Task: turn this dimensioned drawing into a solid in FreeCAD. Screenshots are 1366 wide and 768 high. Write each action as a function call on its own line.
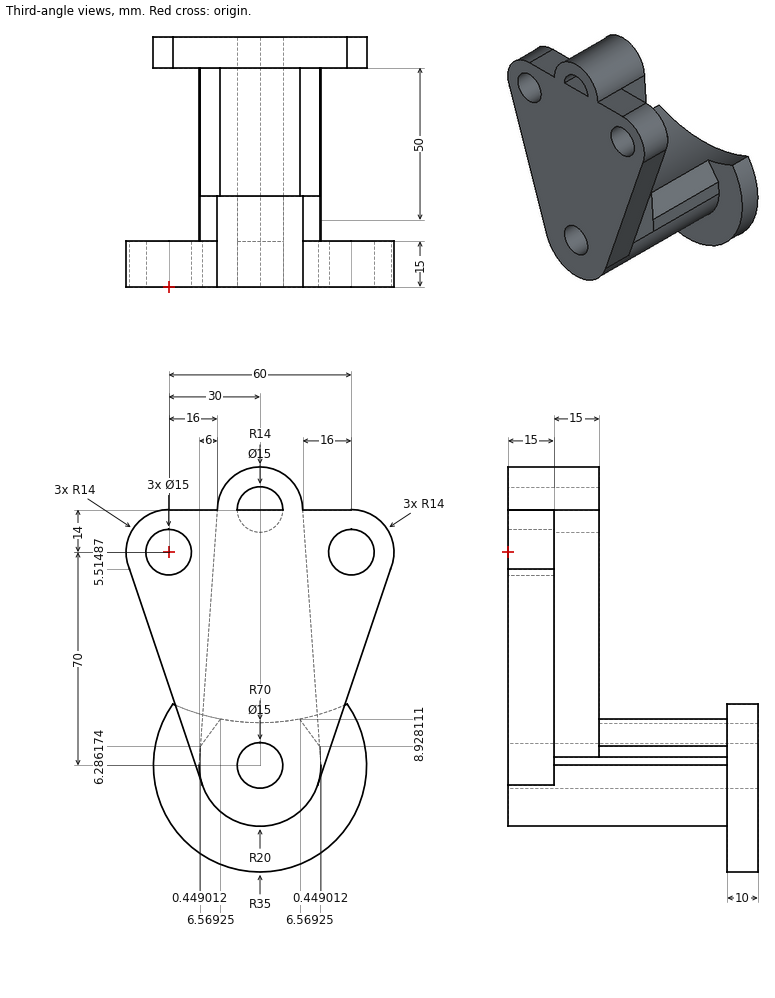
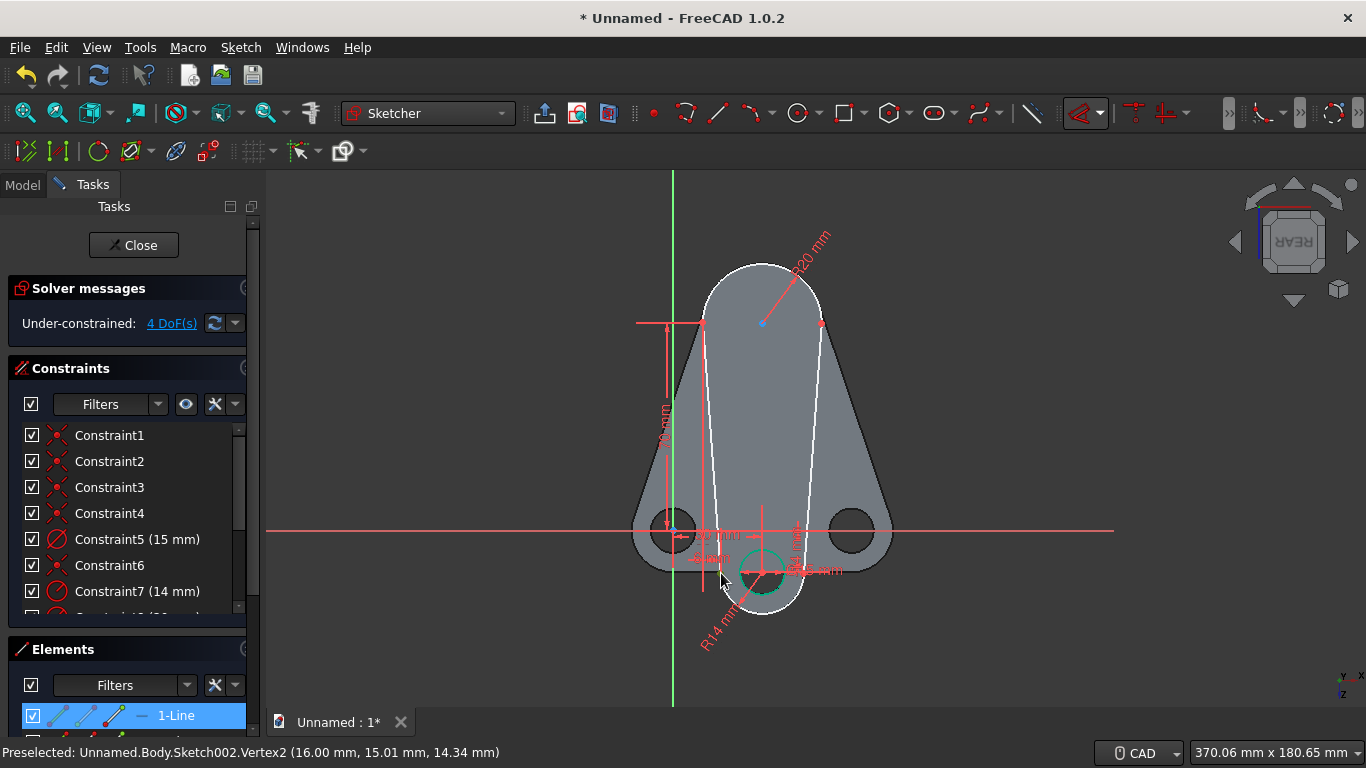
key(i)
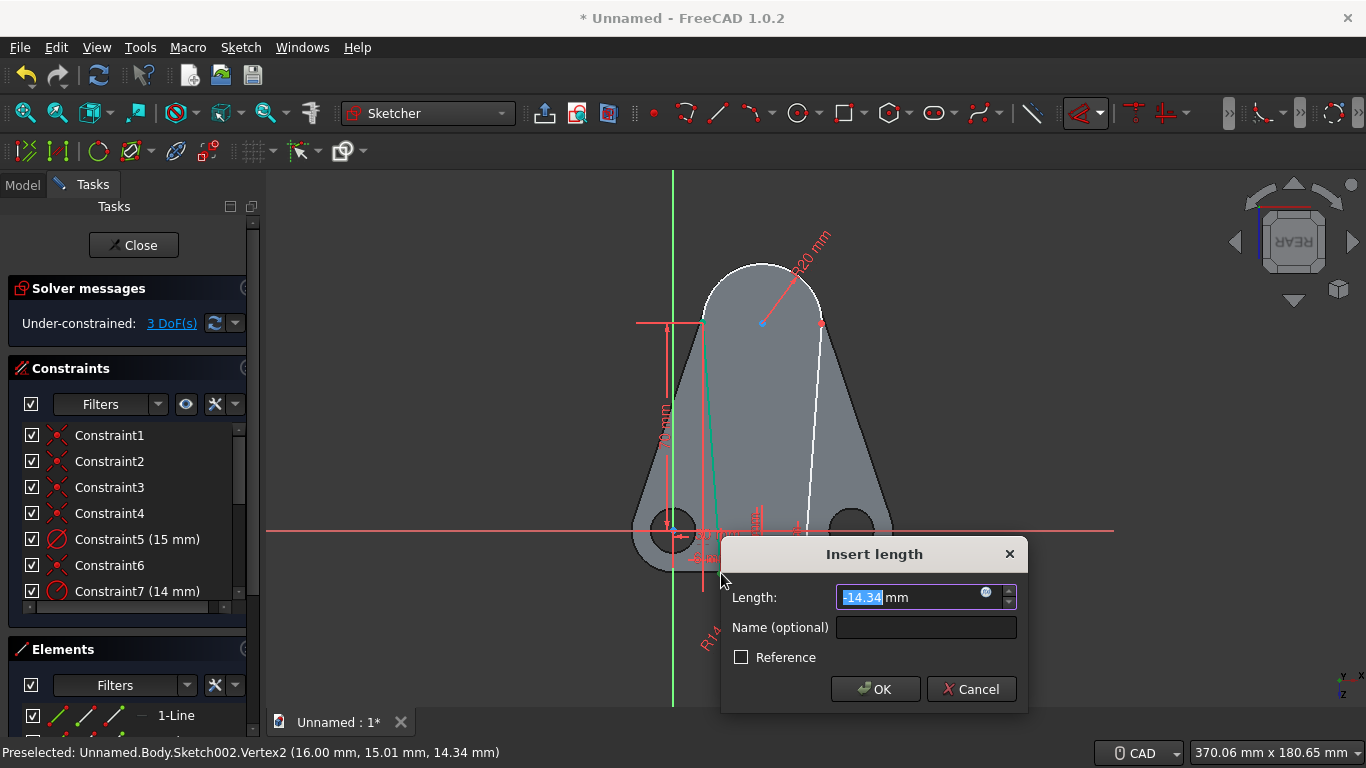
text(-14)
key(Return)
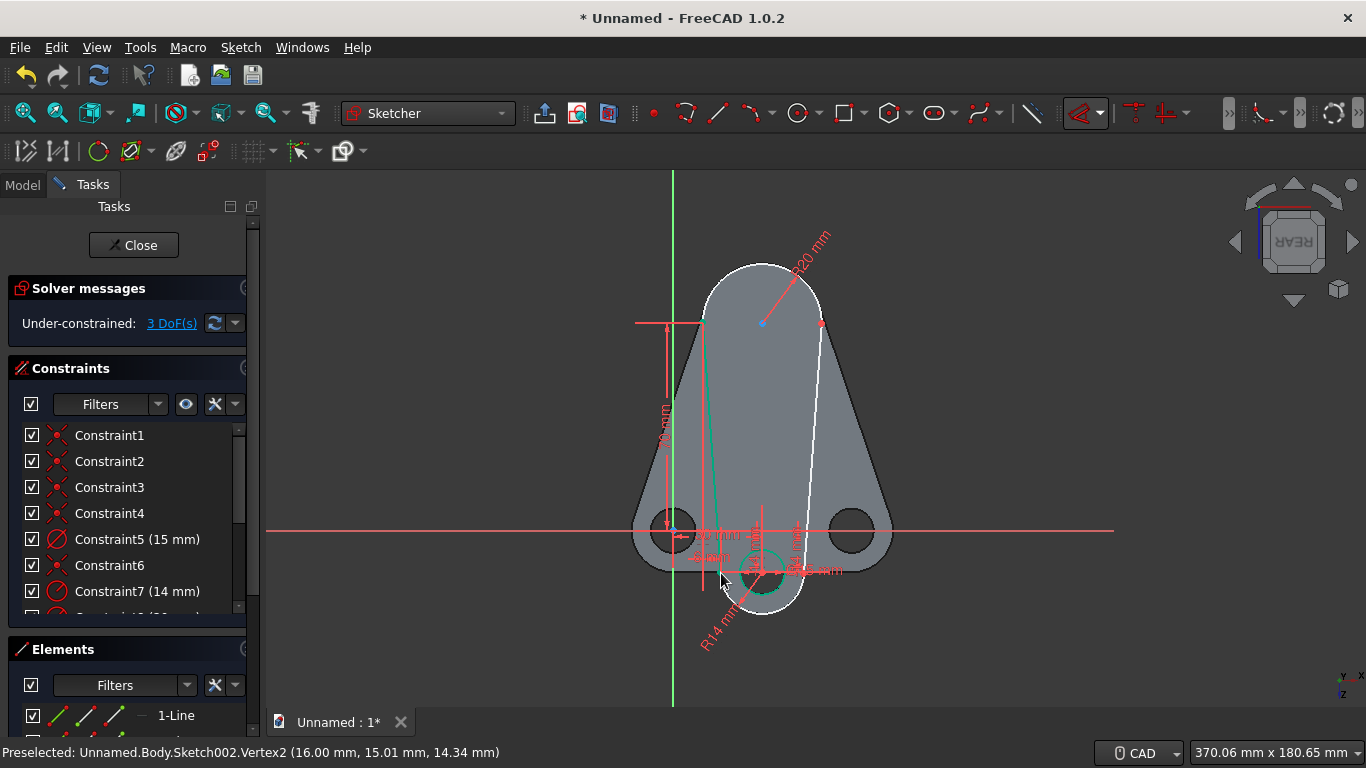
click(804, 573)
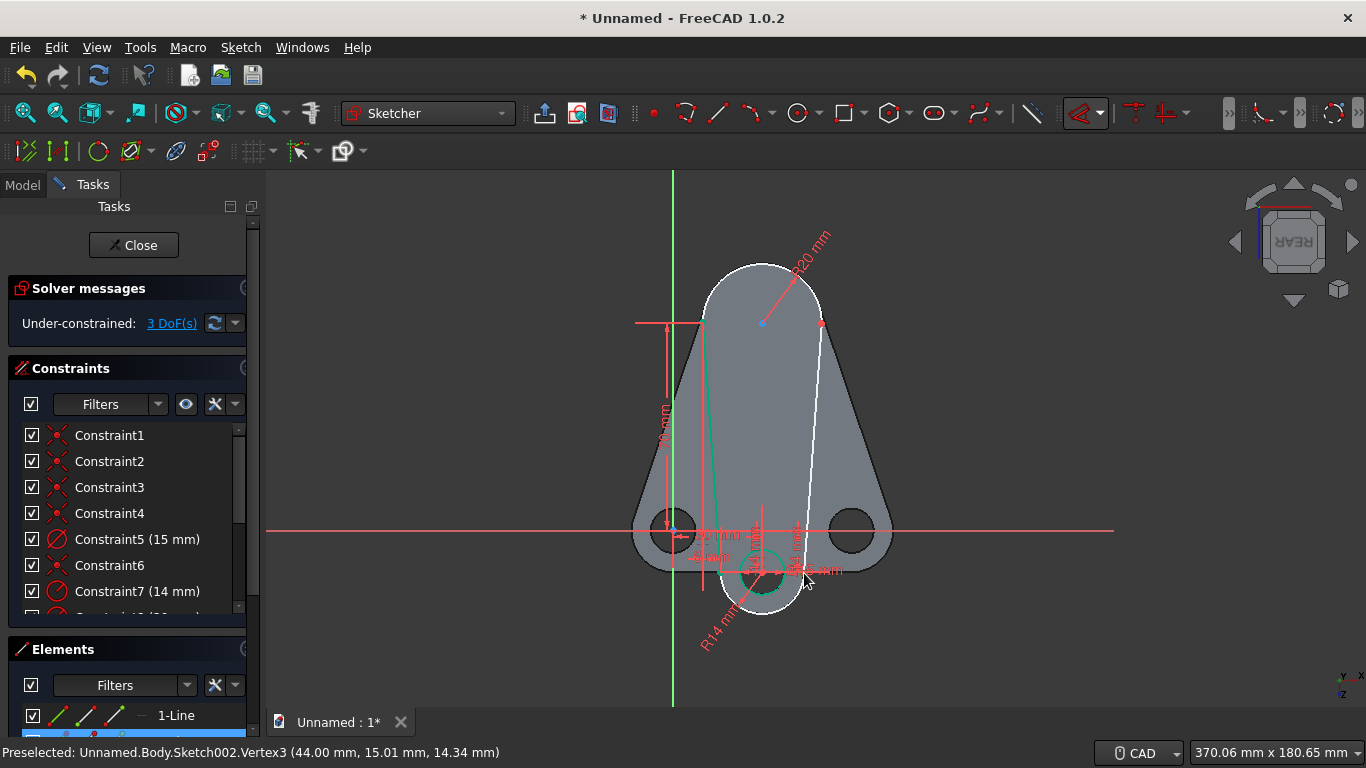
click(1102, 114)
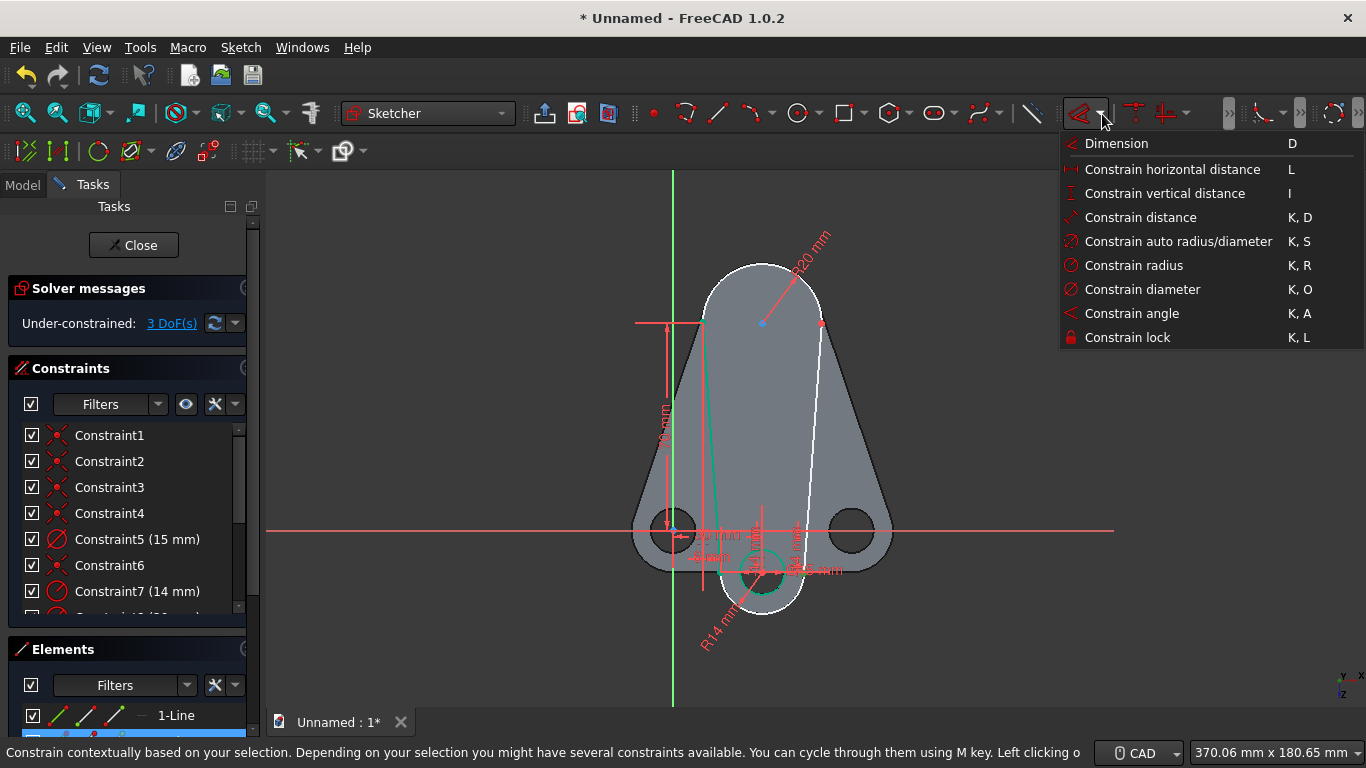
click(1212, 193)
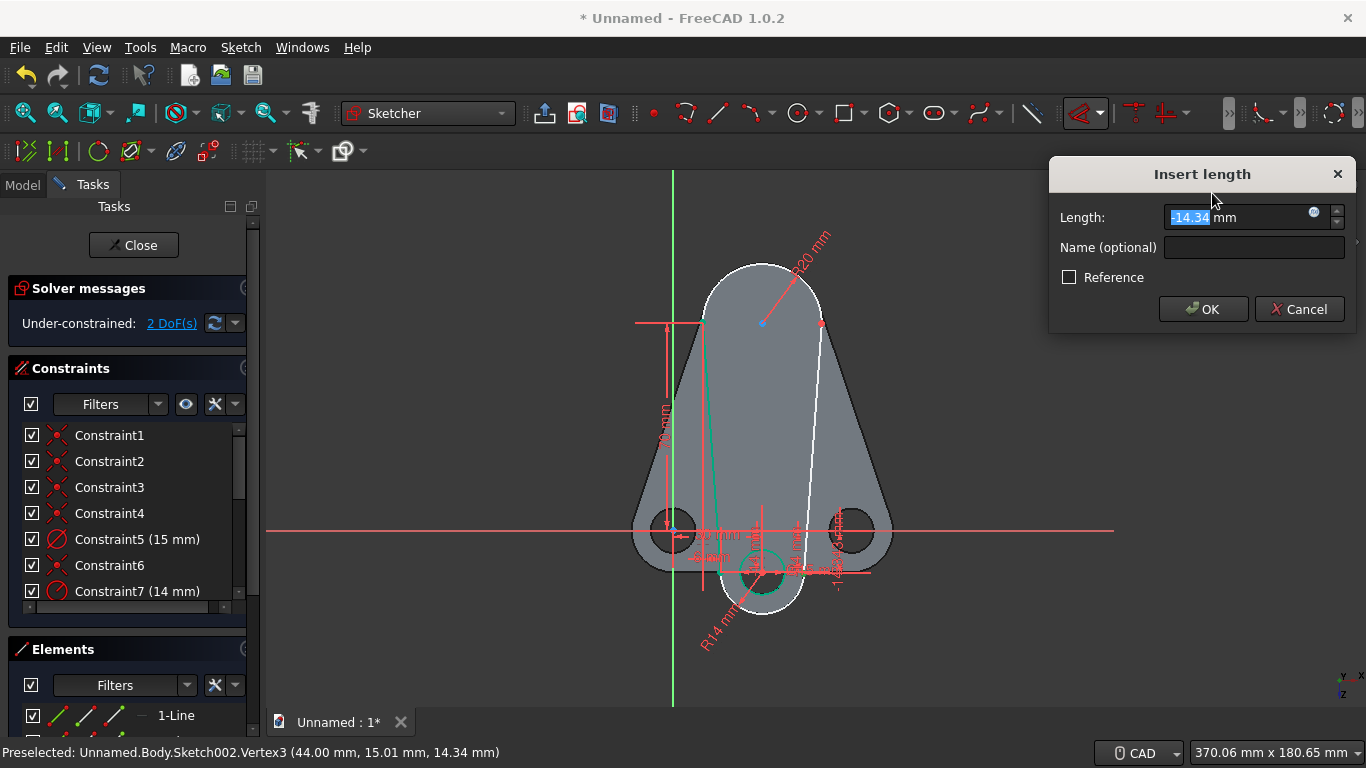
text(-14)
key(Return)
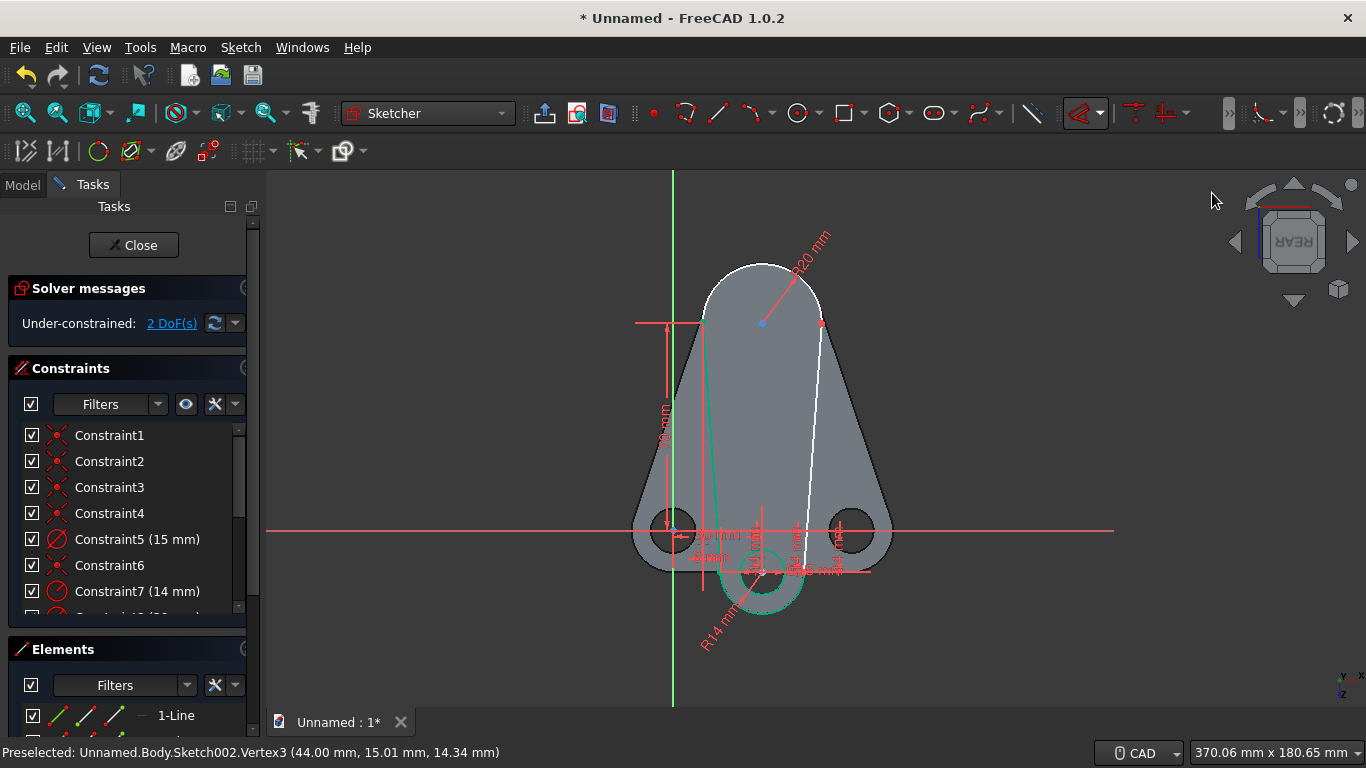
click(822, 324)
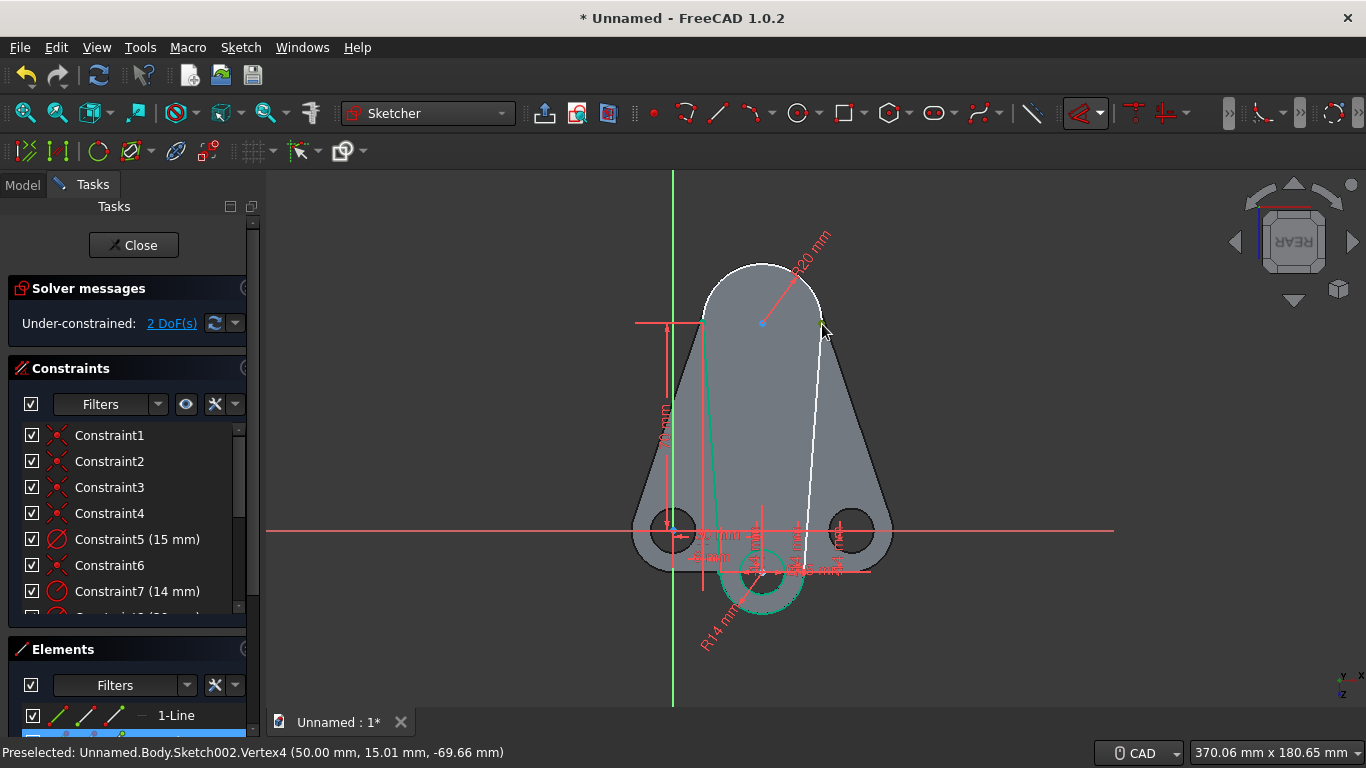
key(i)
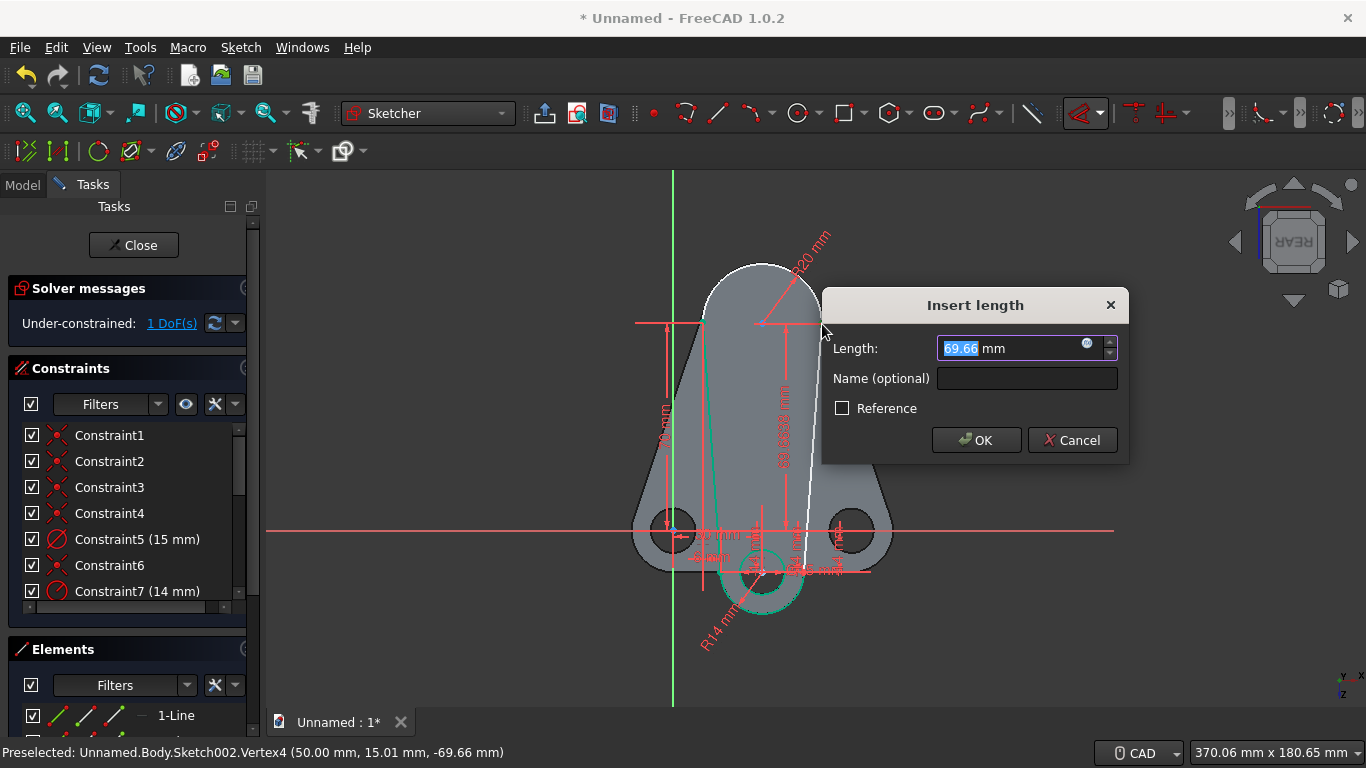
text(70)
key(Return)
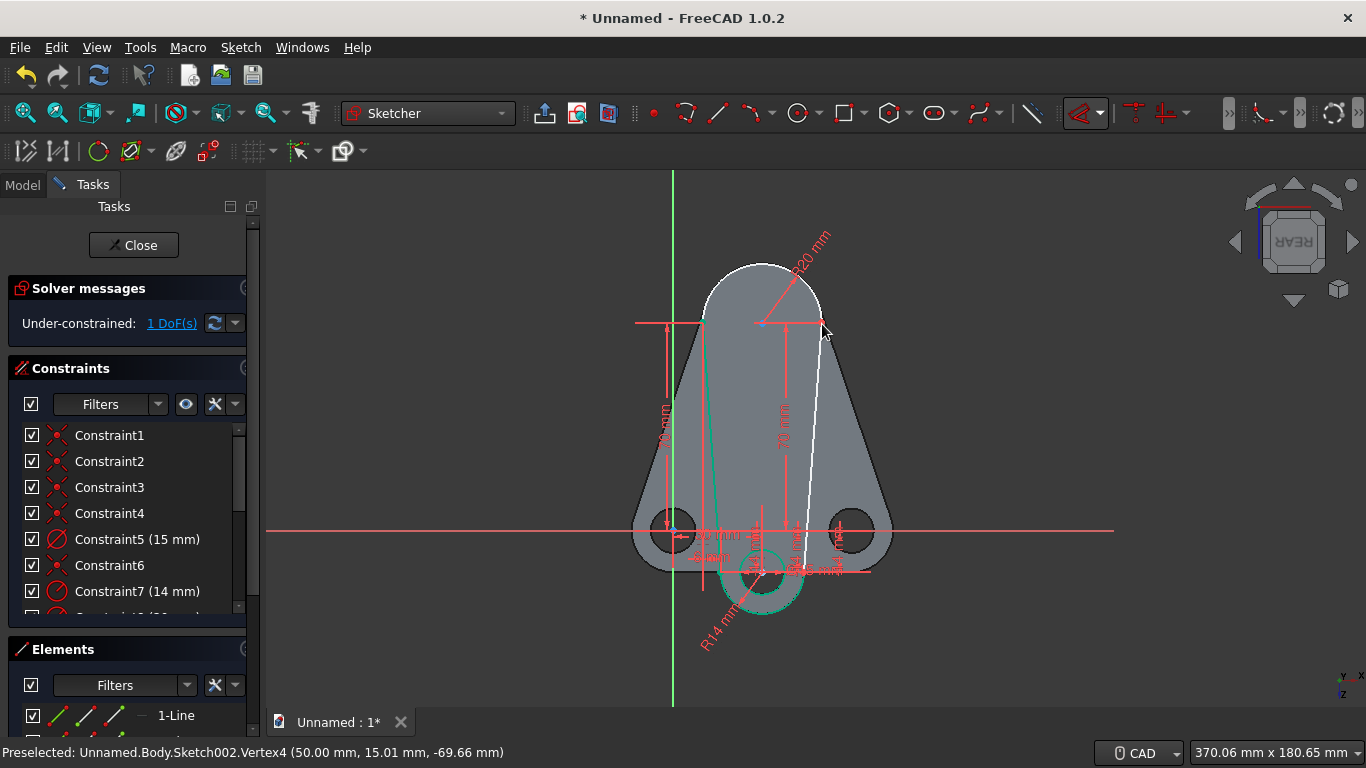
click(762, 324)